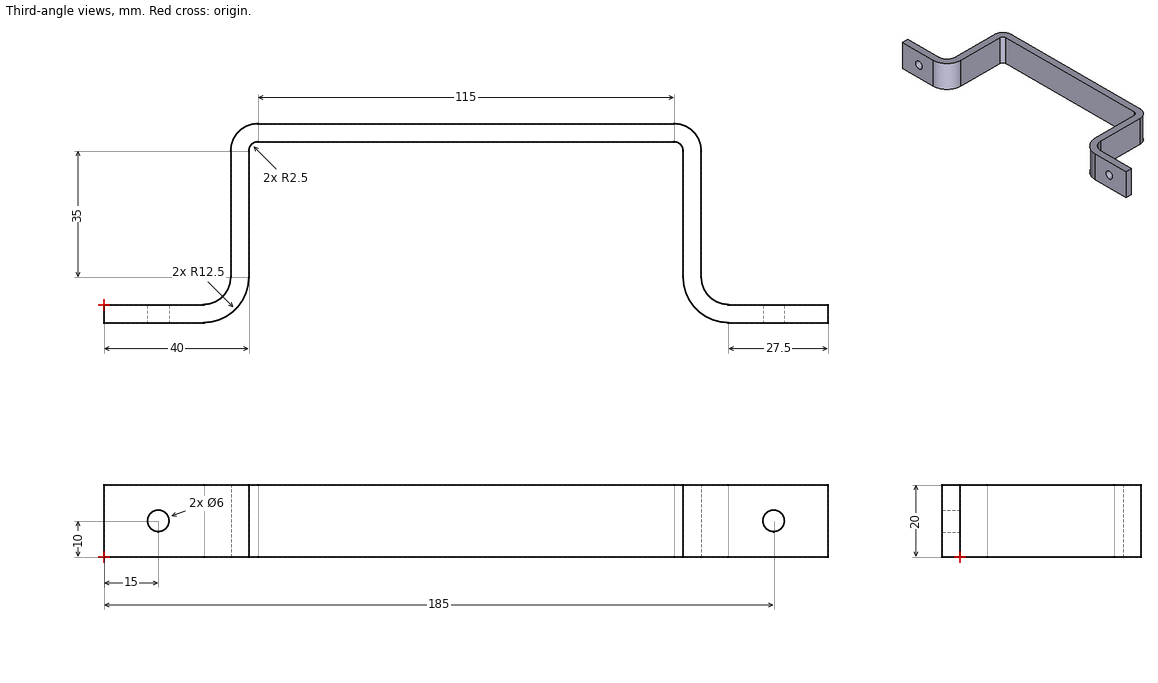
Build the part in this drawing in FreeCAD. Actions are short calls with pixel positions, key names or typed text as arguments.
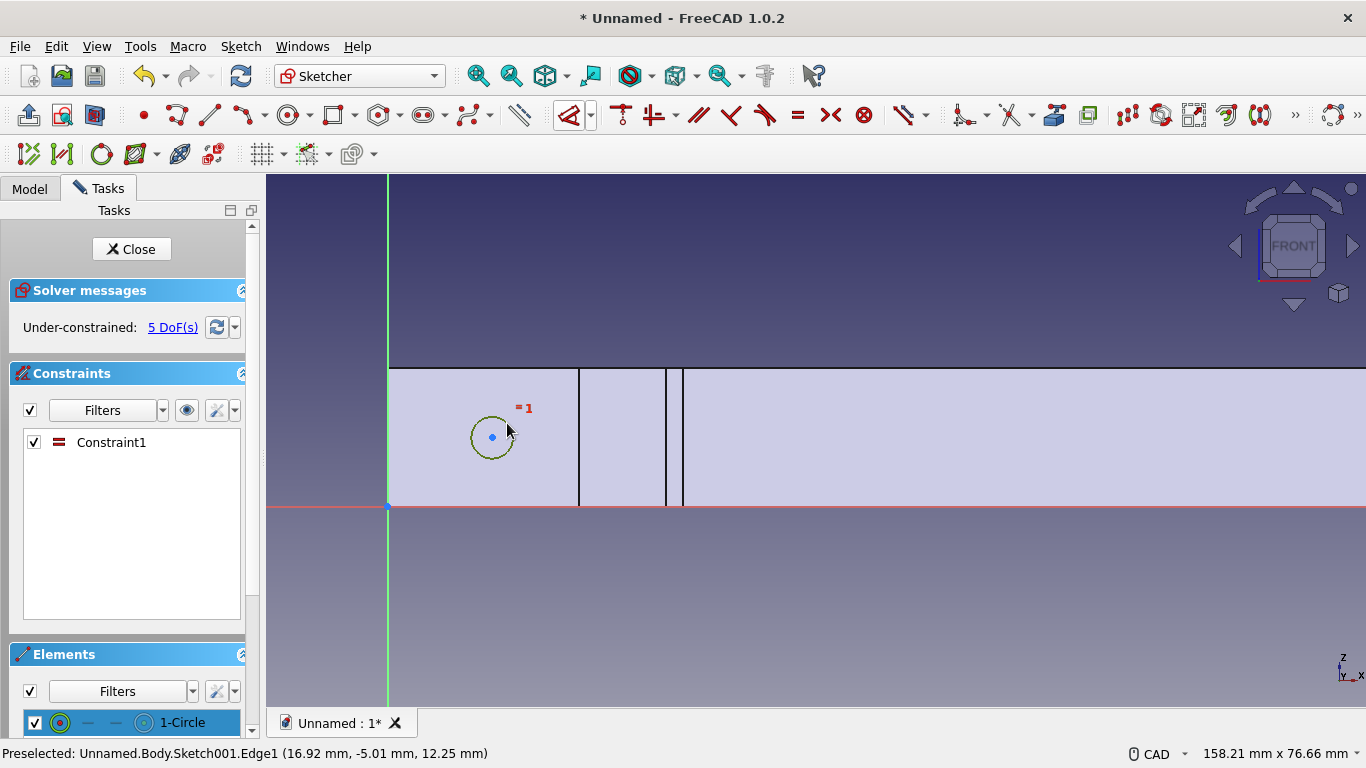
click(590, 116)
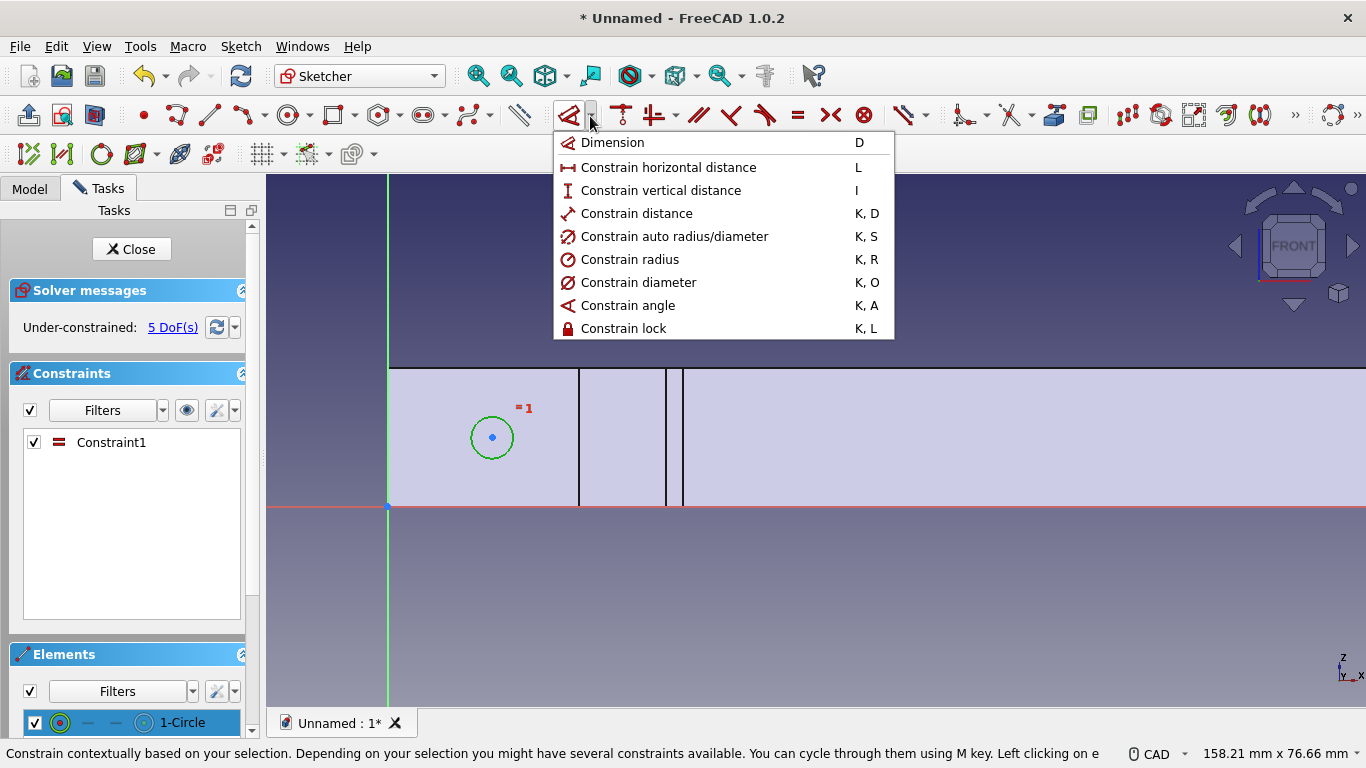
click(724, 282)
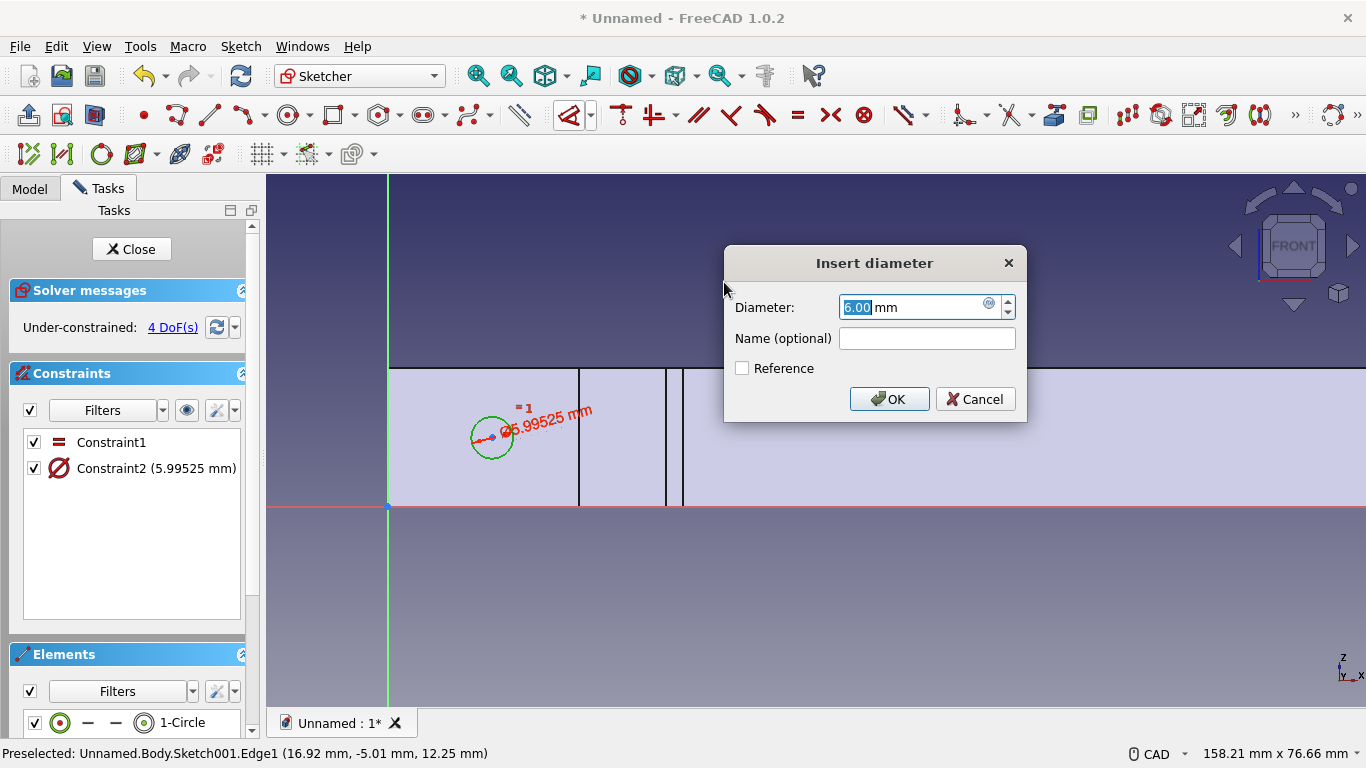
text(6)
key(Return)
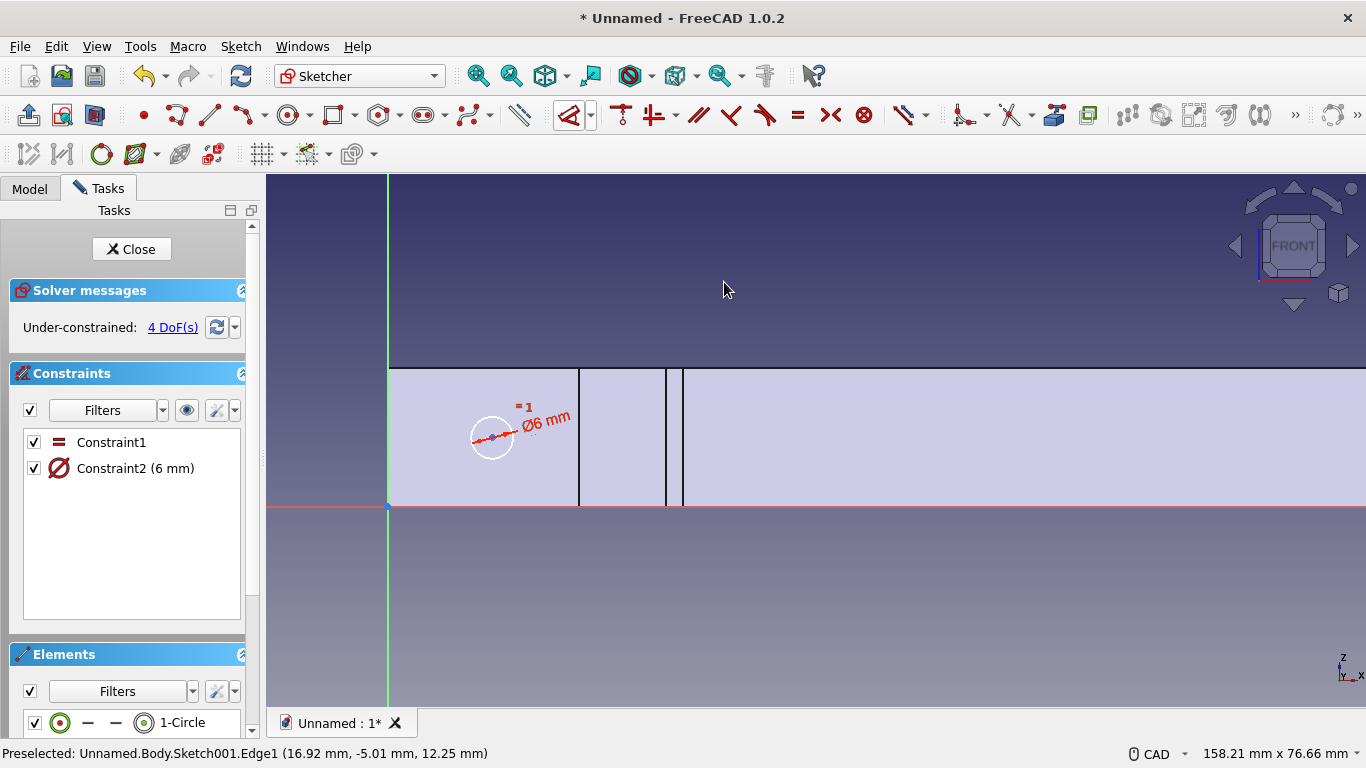
click(492, 438)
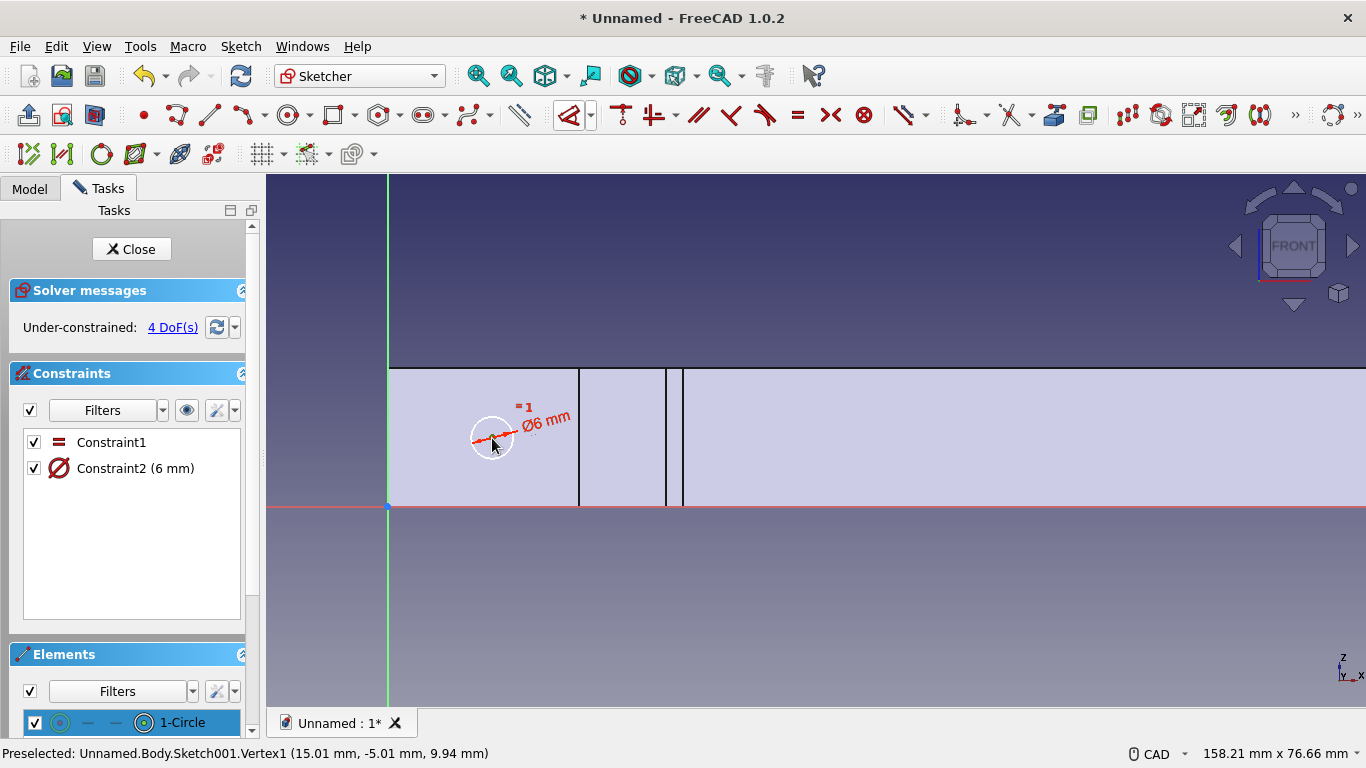
key(l)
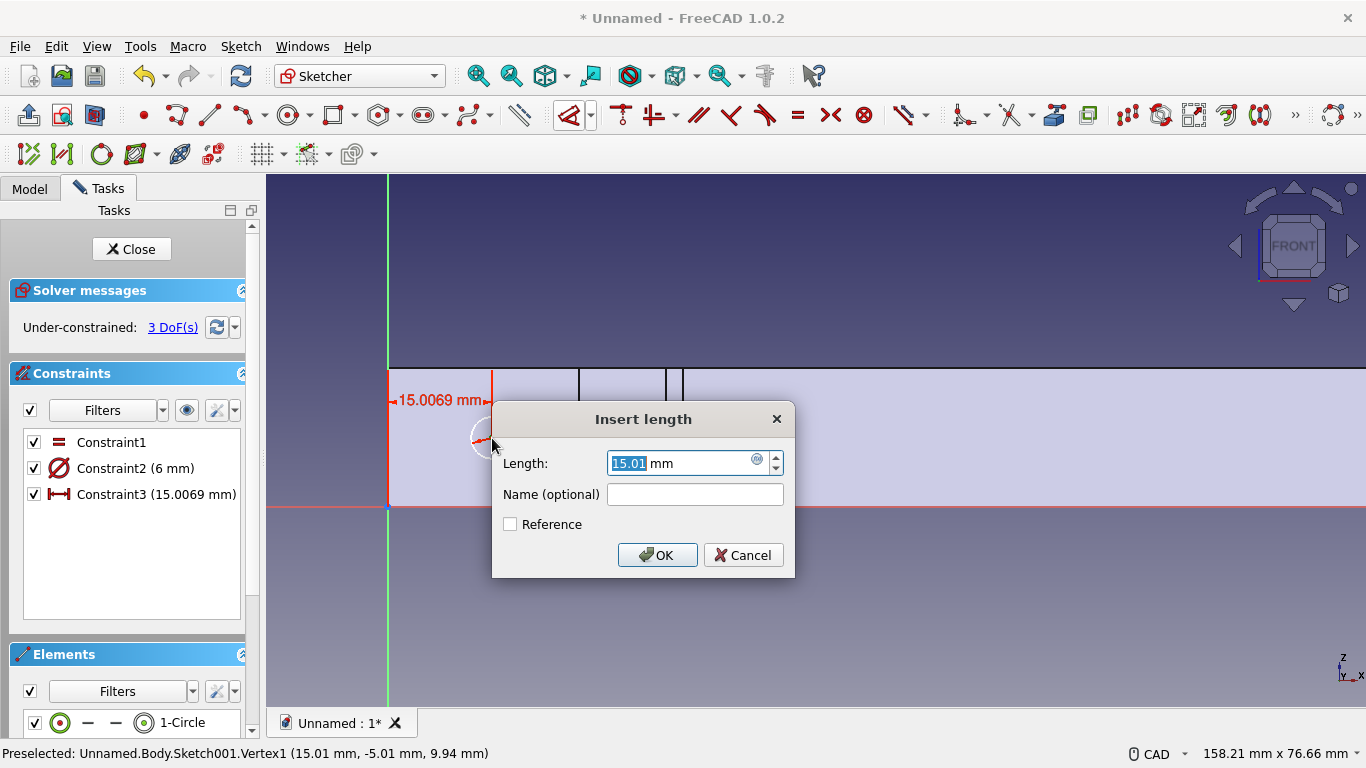
text(15)
key(Return)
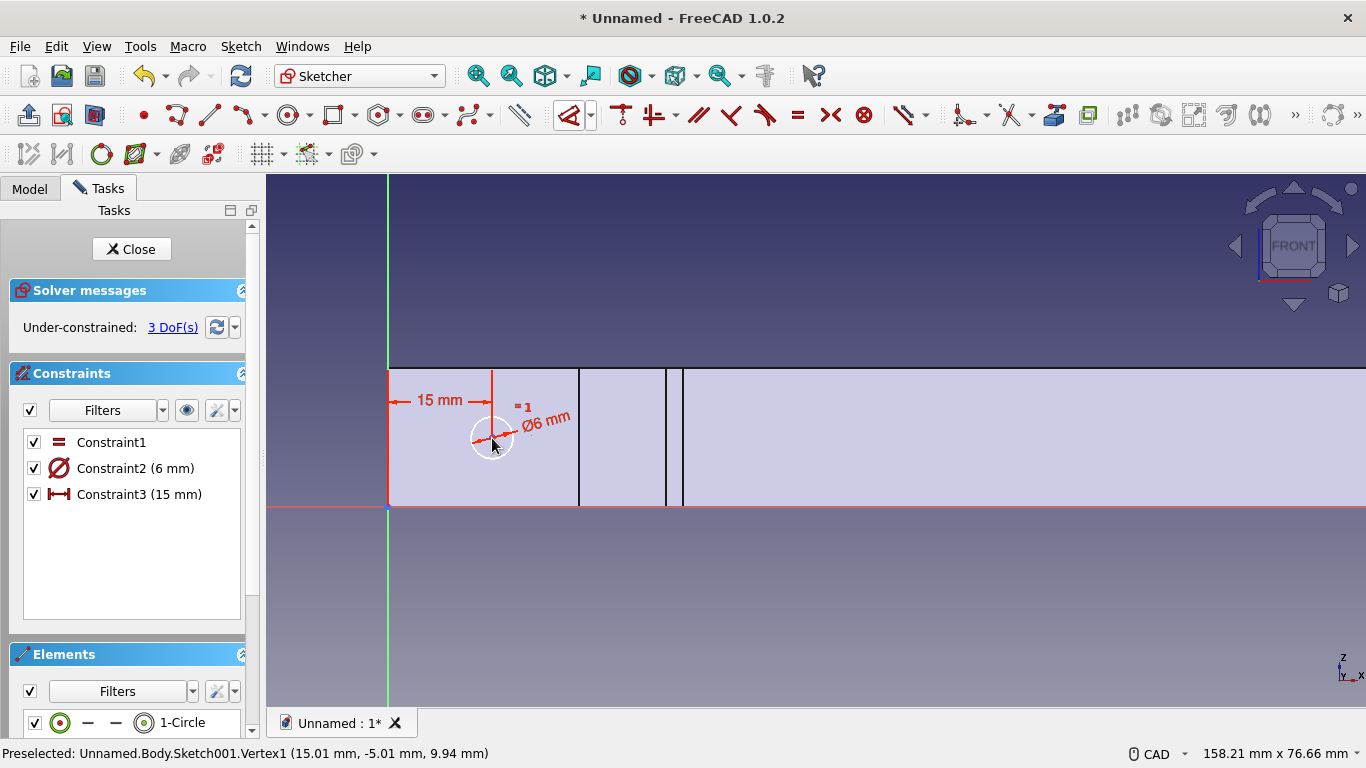
click(492, 438)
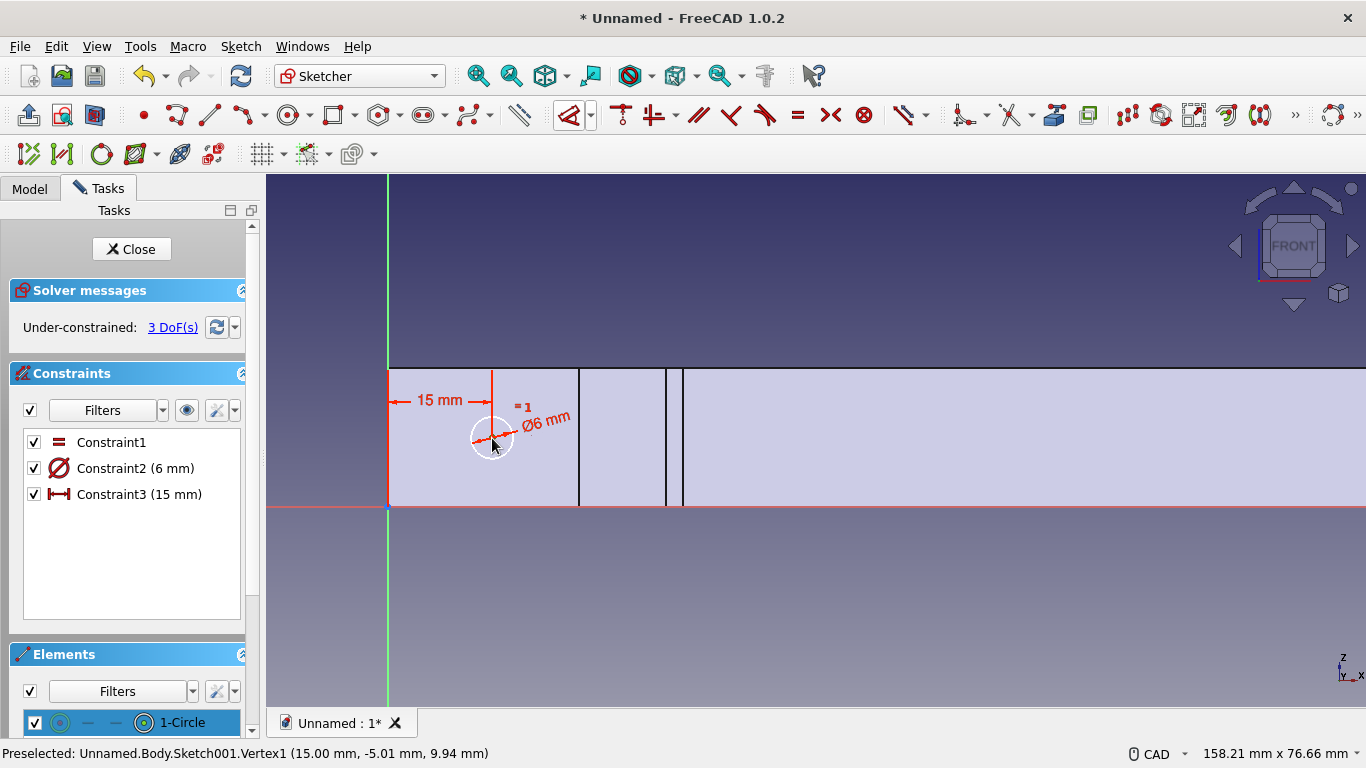
key(i)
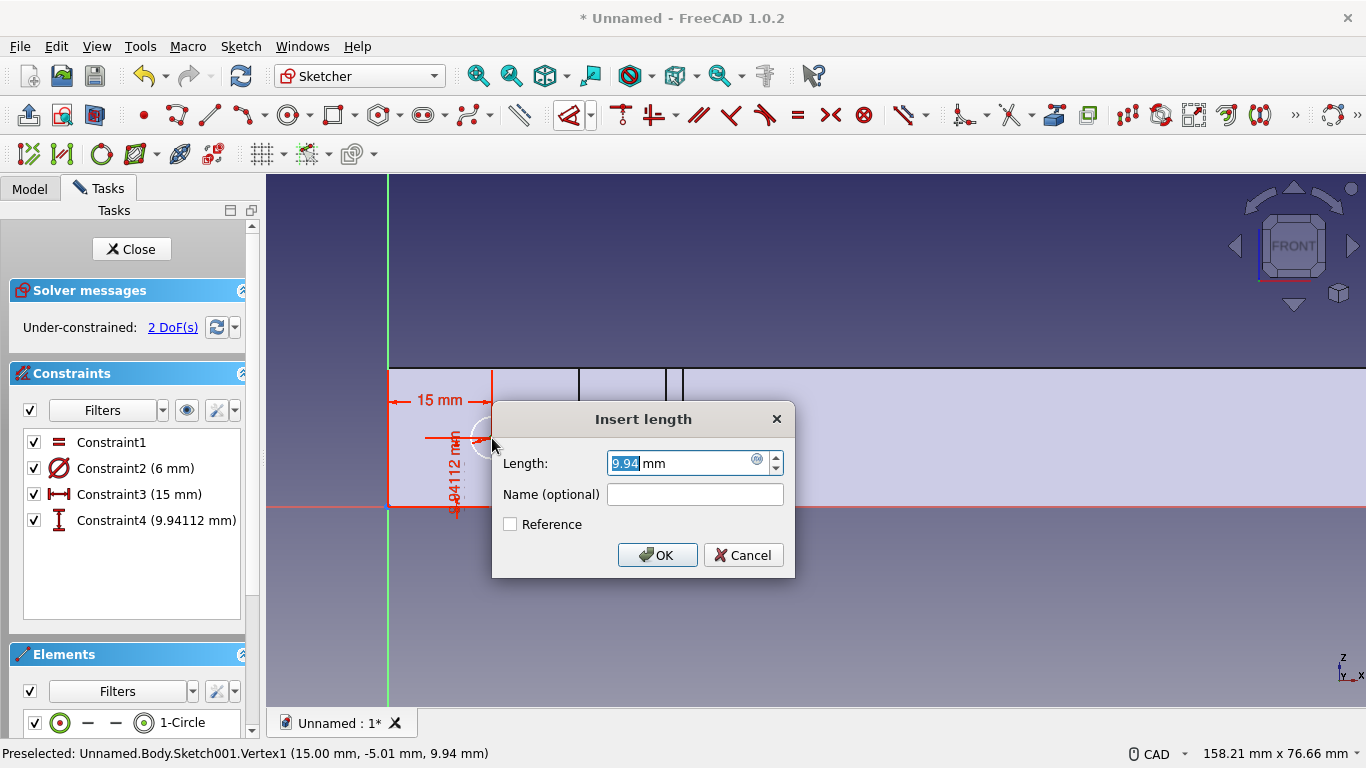
text(10)
key(Return)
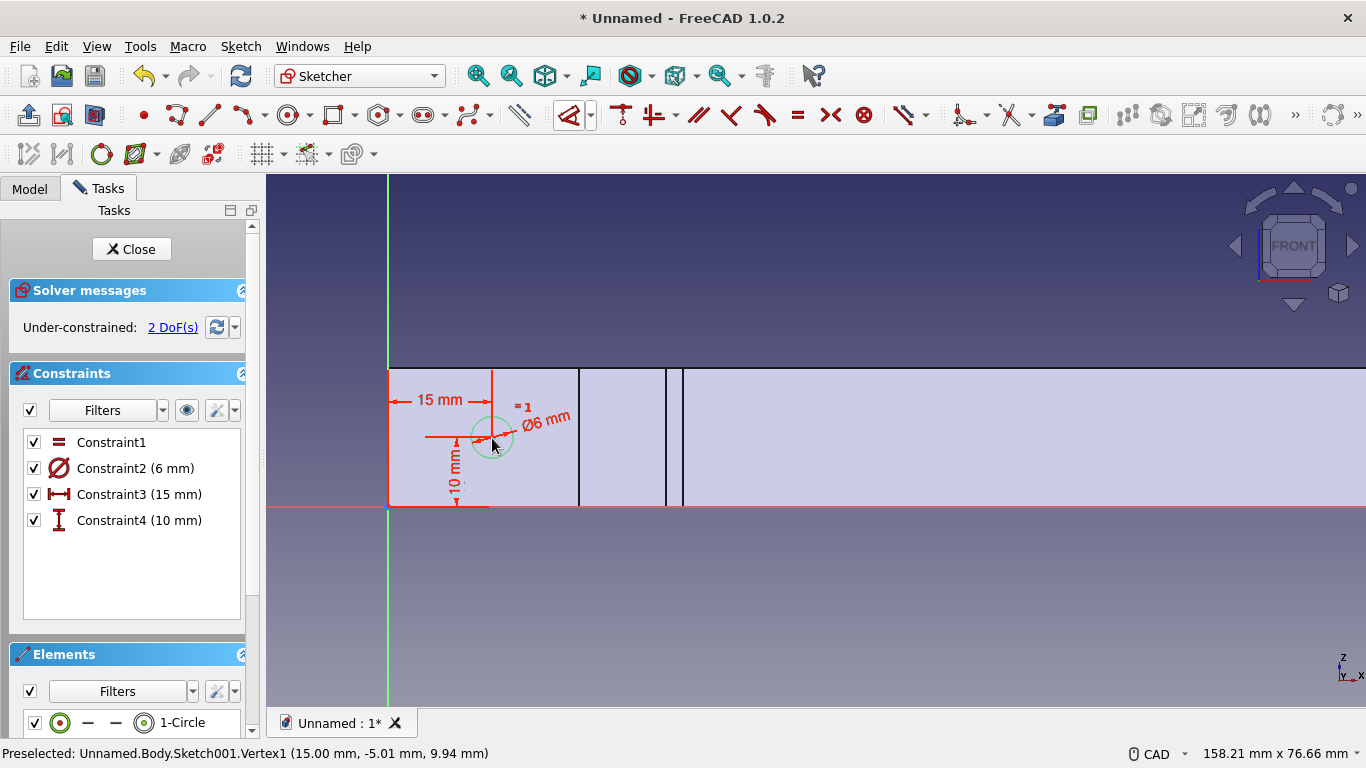
scroll(508, 423, down, 4)